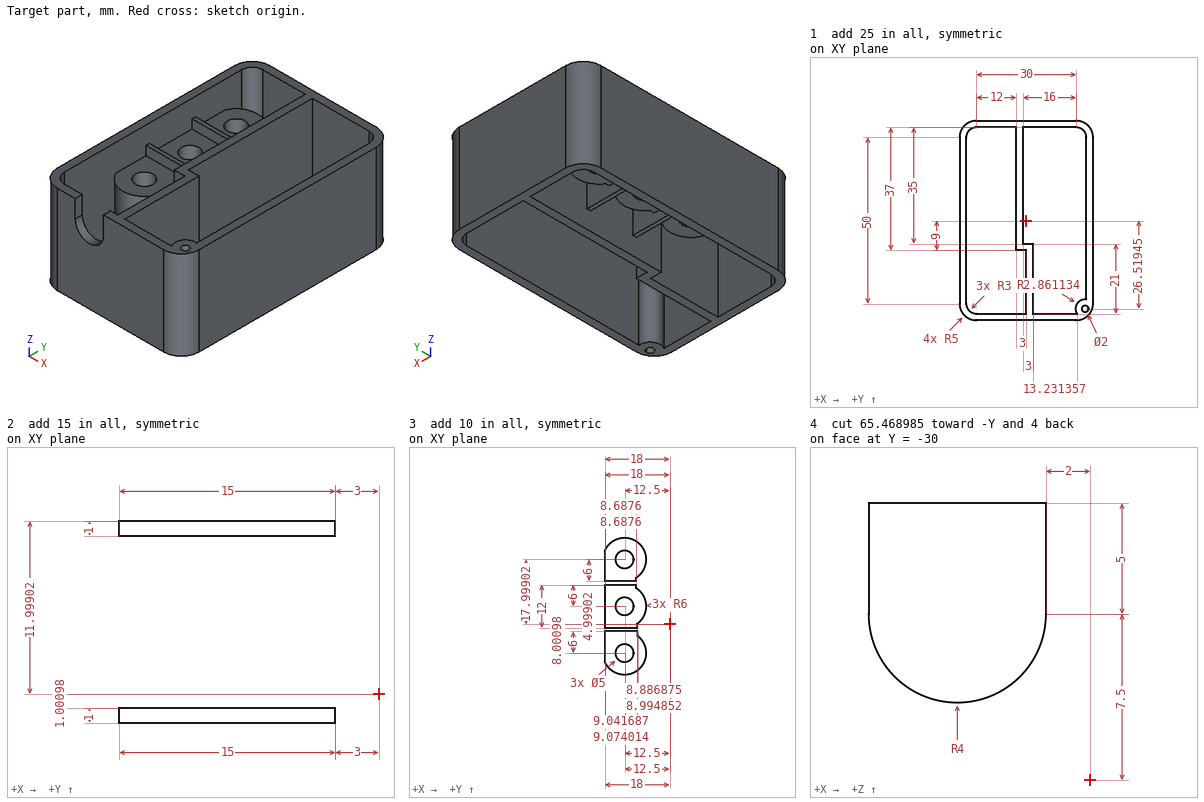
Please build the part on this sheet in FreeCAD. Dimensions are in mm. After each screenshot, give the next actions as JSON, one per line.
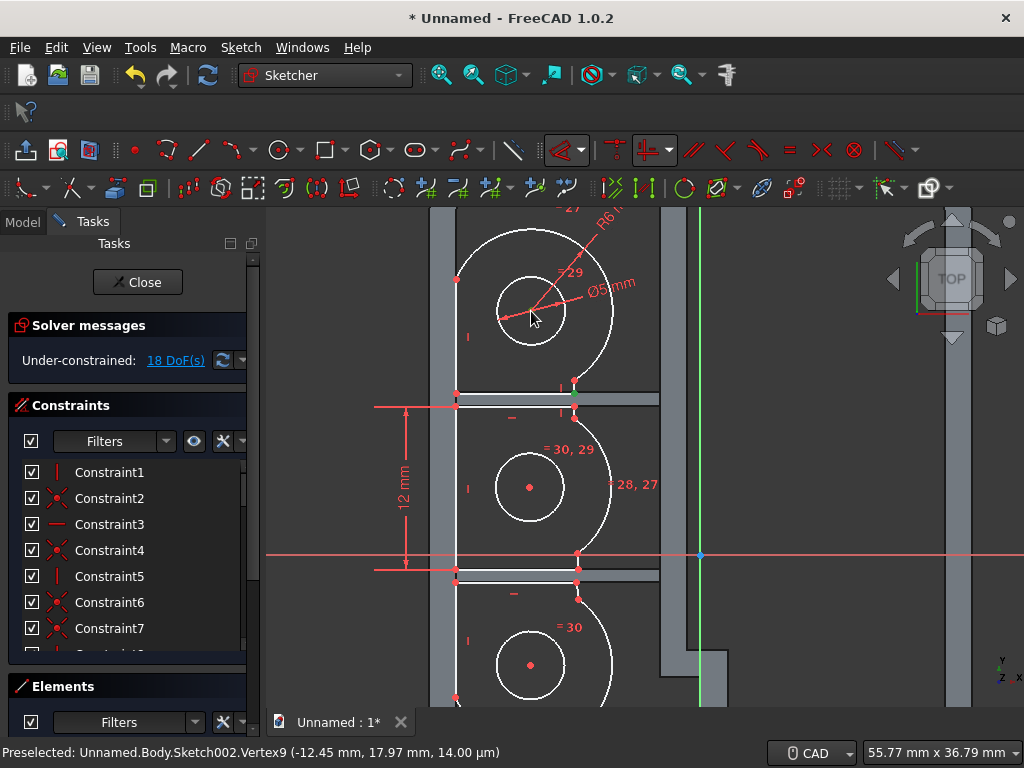
{"action": "left_click", "coordinate": [584, 150]}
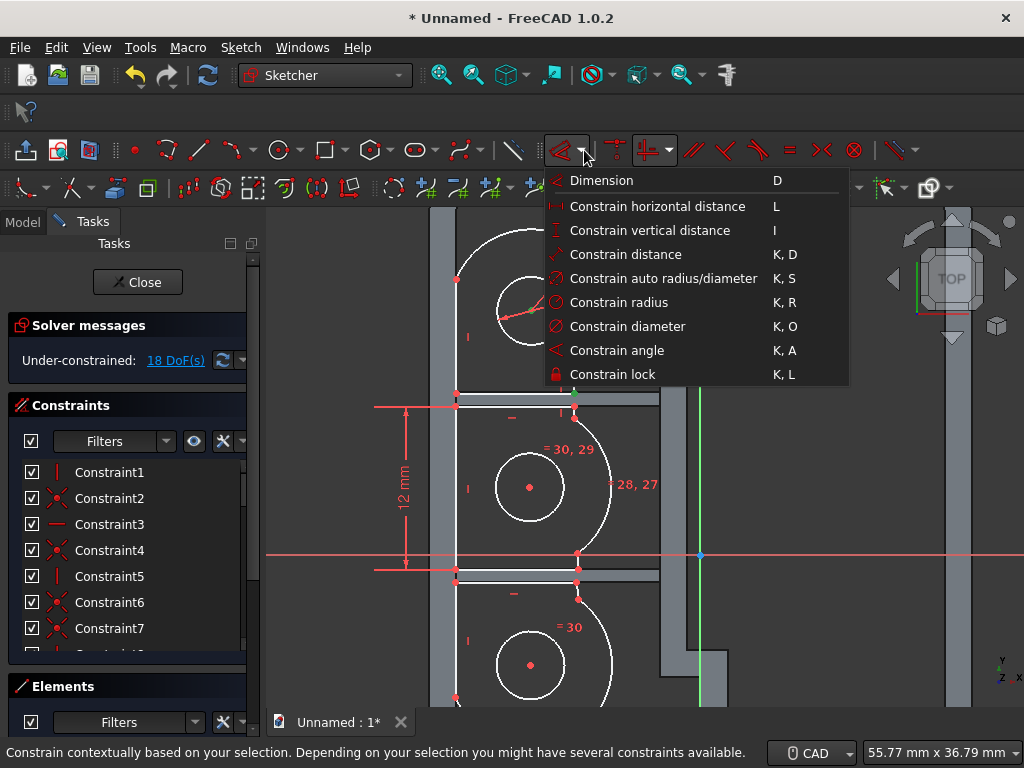
{"action": "left_click", "coordinate": [697, 230]}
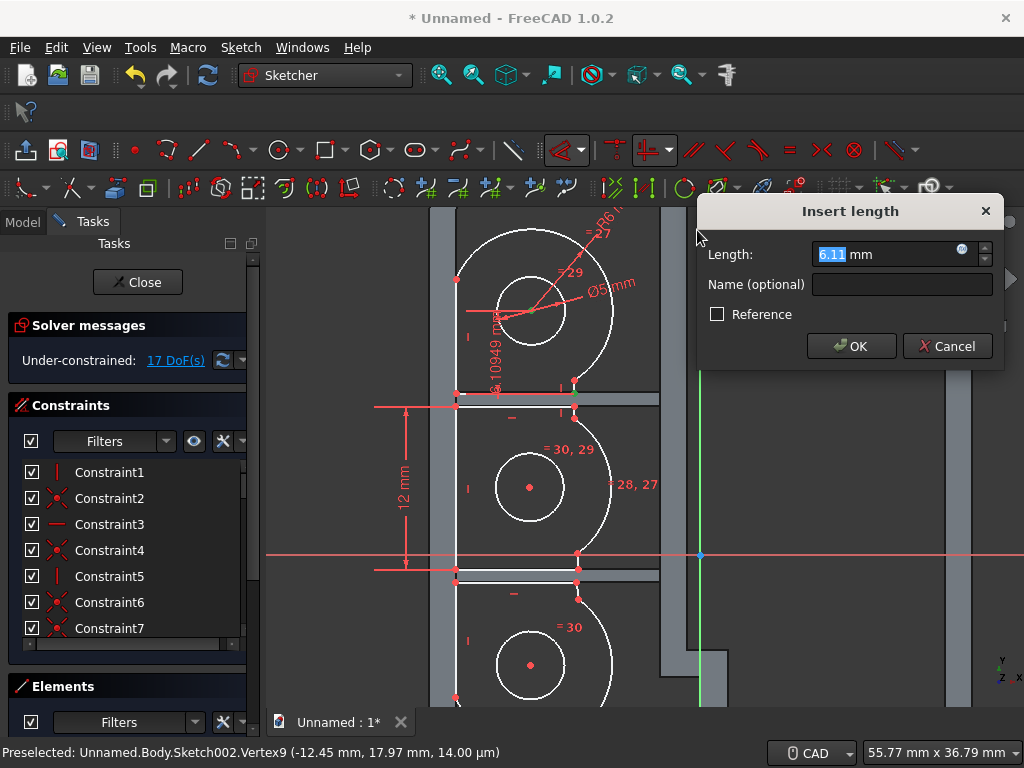
{"action": "type", "text": "6"}
{"action": "key", "text": "Return"}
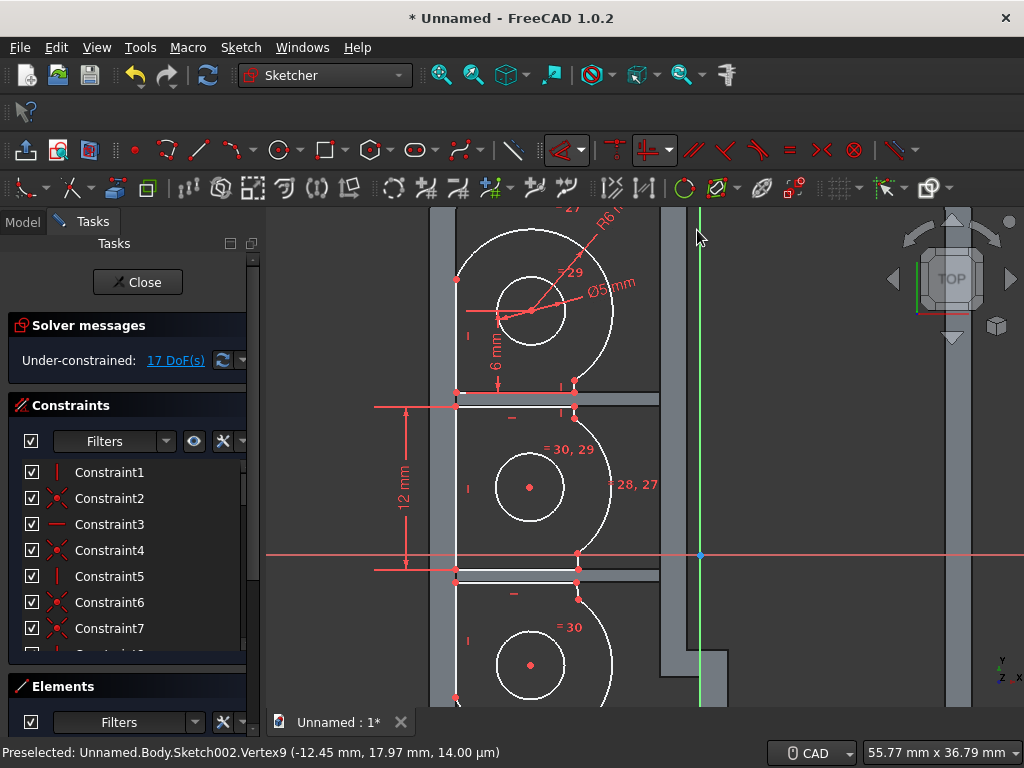
{"action": "left_click", "coordinate": [574, 407]}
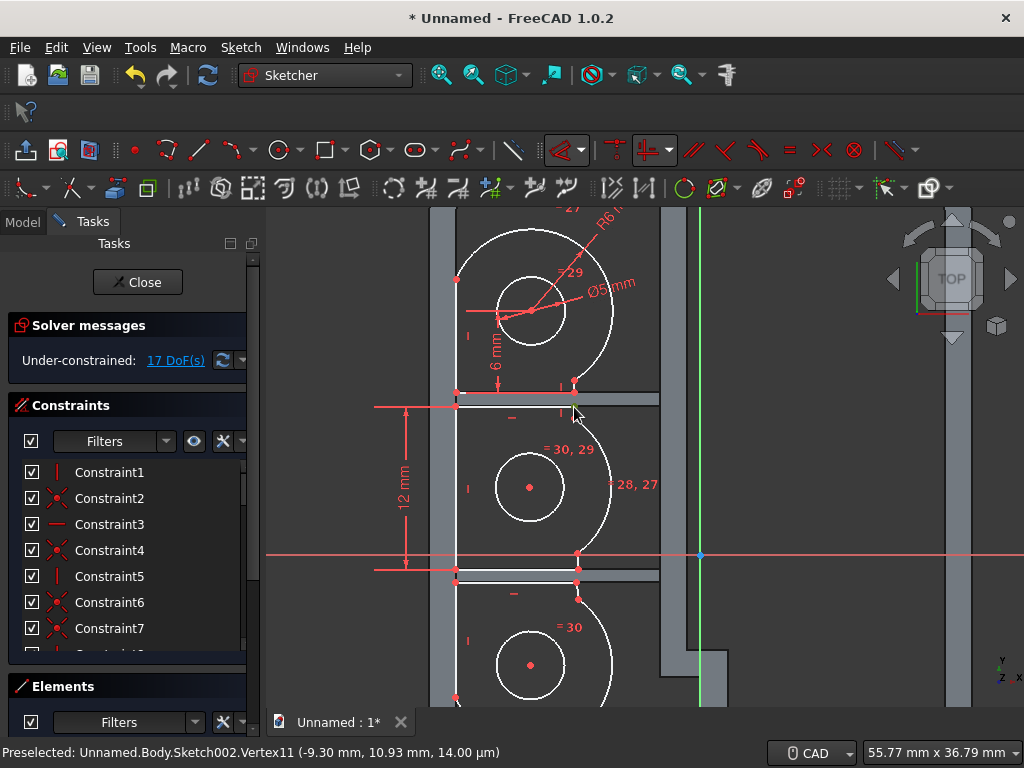
{"action": "left_click", "coordinate": [530, 487]}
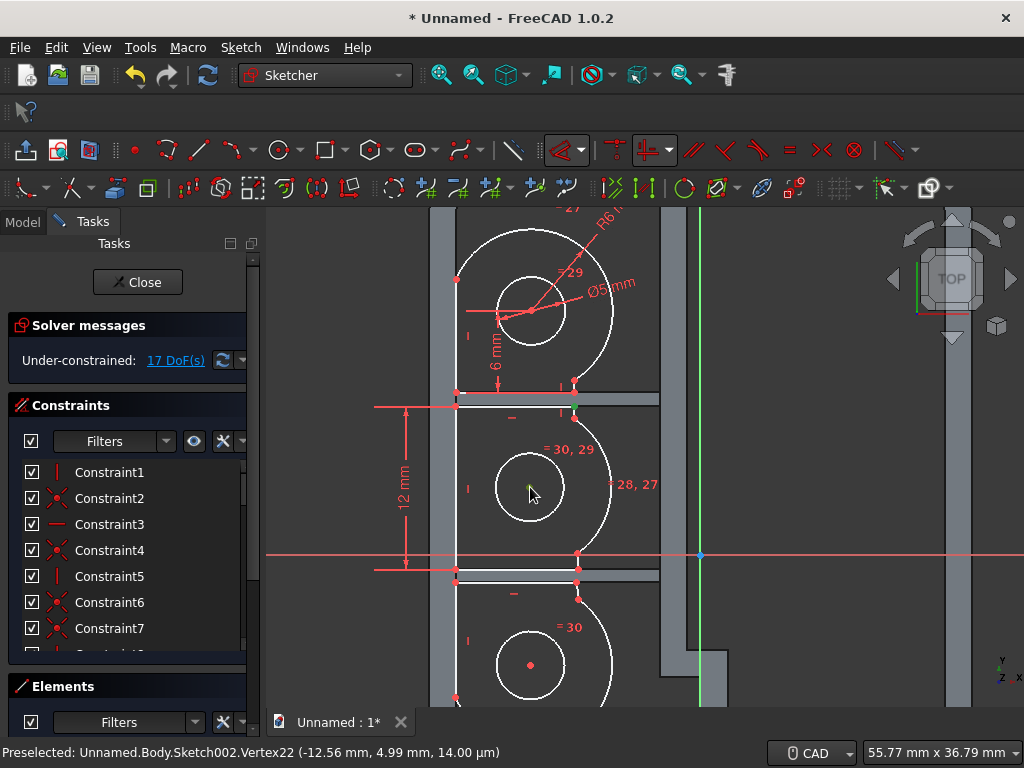
{"action": "left_click", "coordinate": [584, 150]}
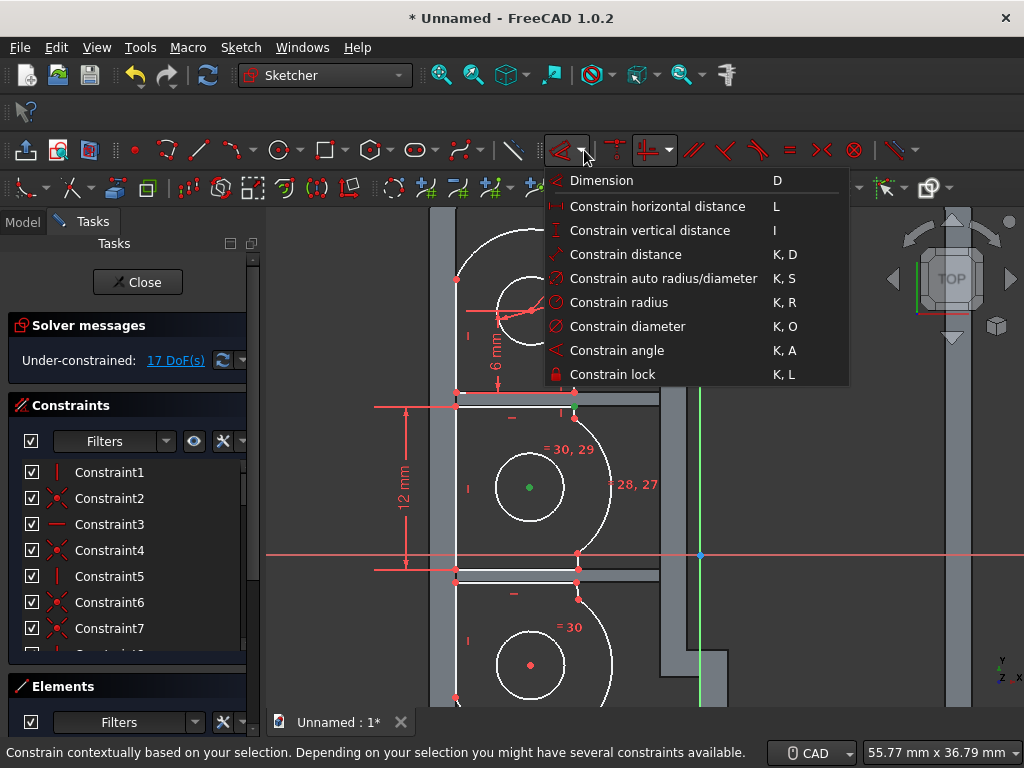
{"action": "left_click", "coordinate": [697, 230]}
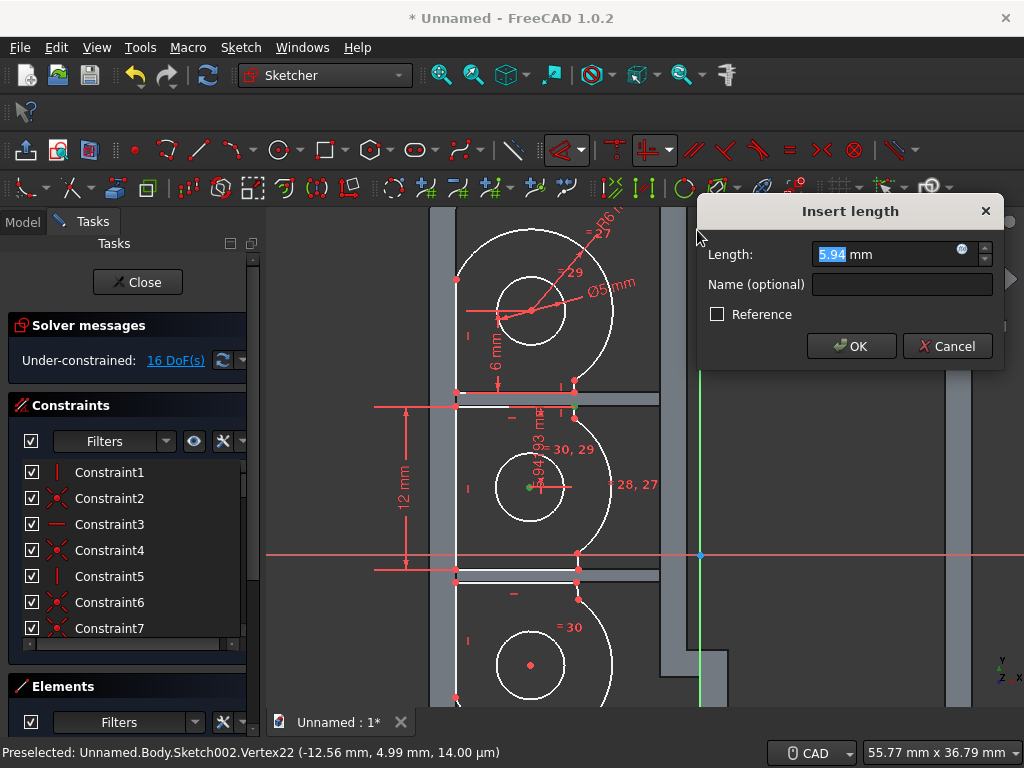
{"action": "type", "text": "6"}
{"action": "key", "text": "Return"}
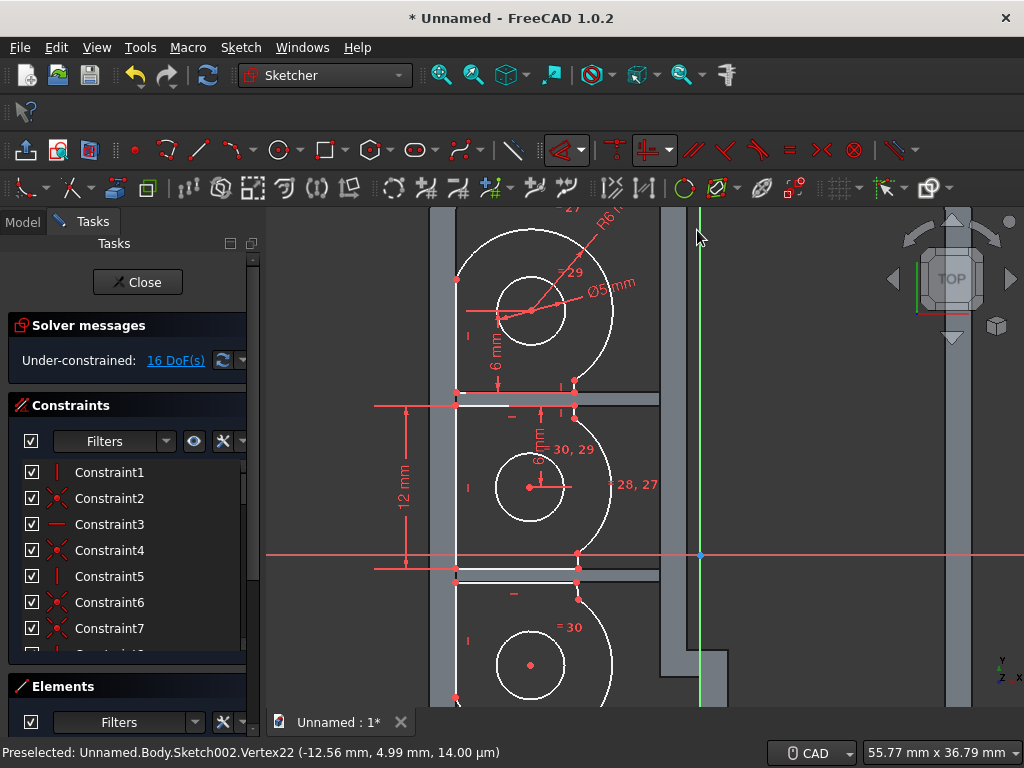
{"action": "left_click", "coordinate": [577, 583]}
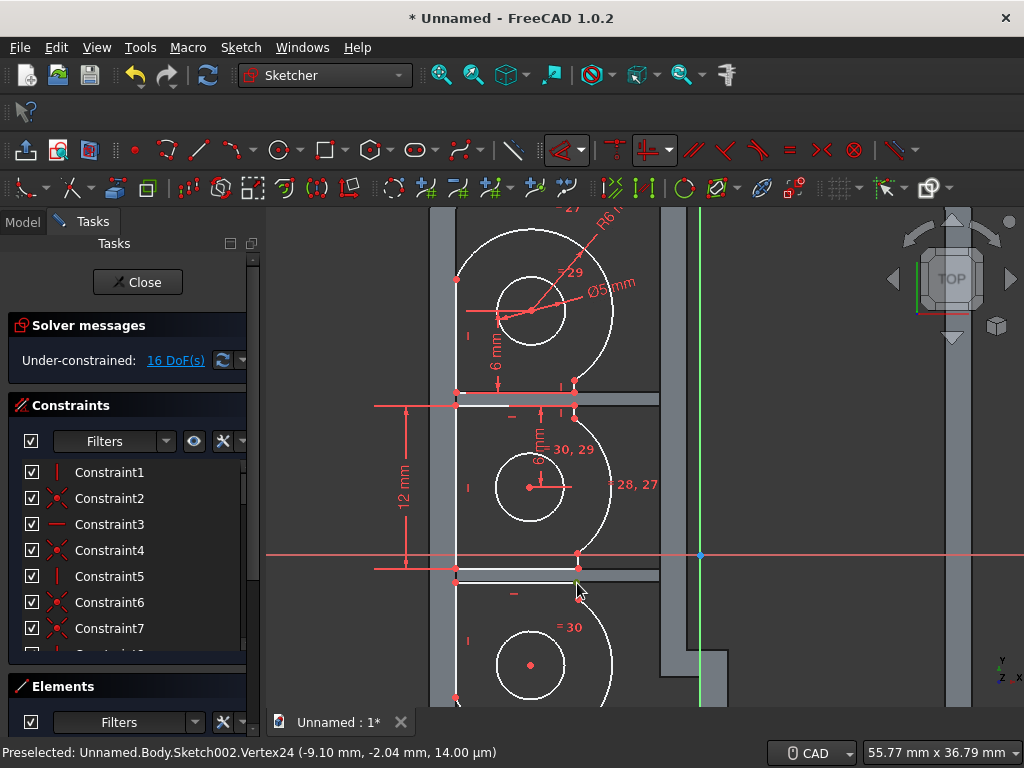
{"action": "left_click", "coordinate": [531, 665]}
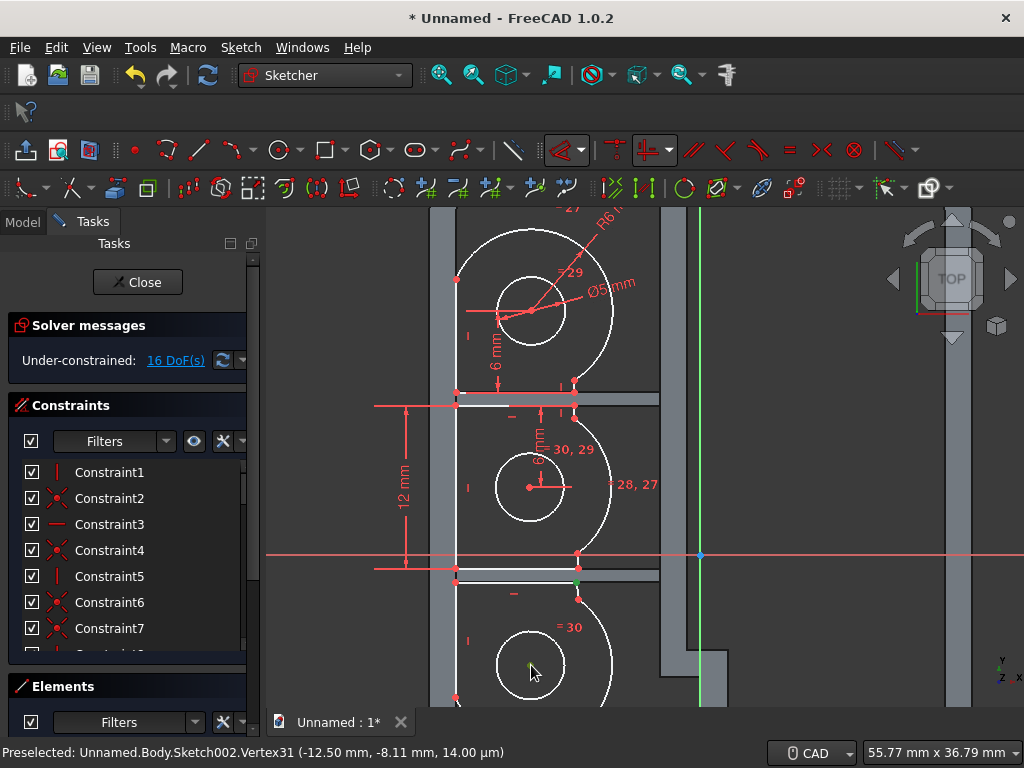
{"action": "key", "text": "i"}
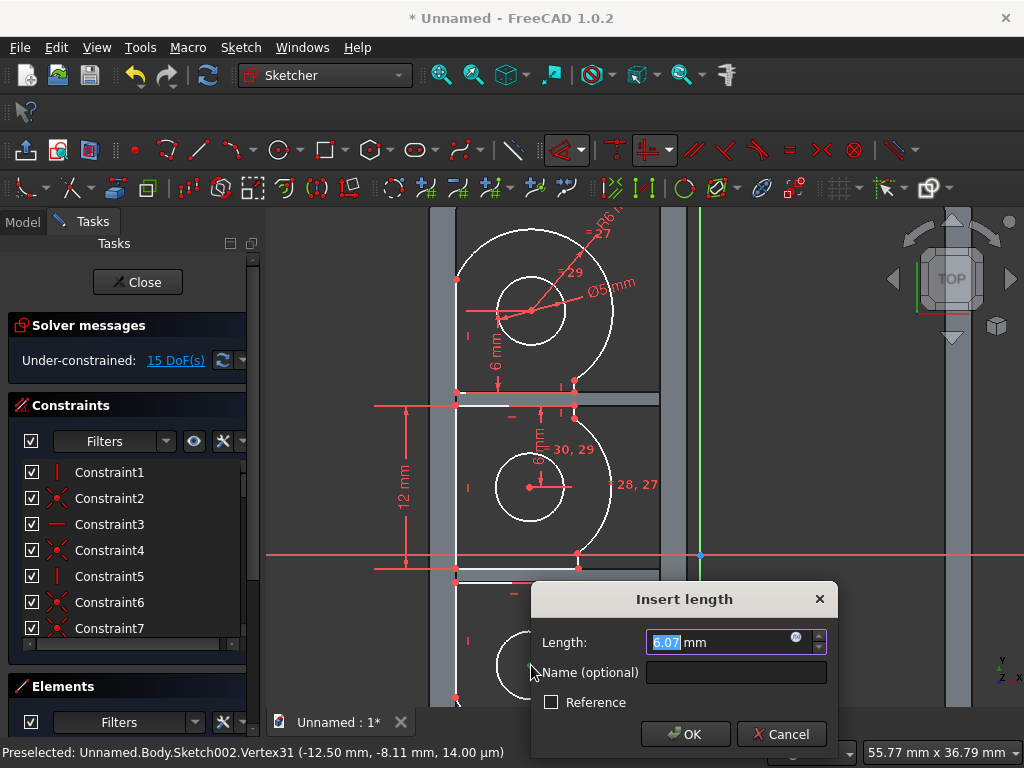
{"action": "type", "text": "6"}
{"action": "key", "text": "Return"}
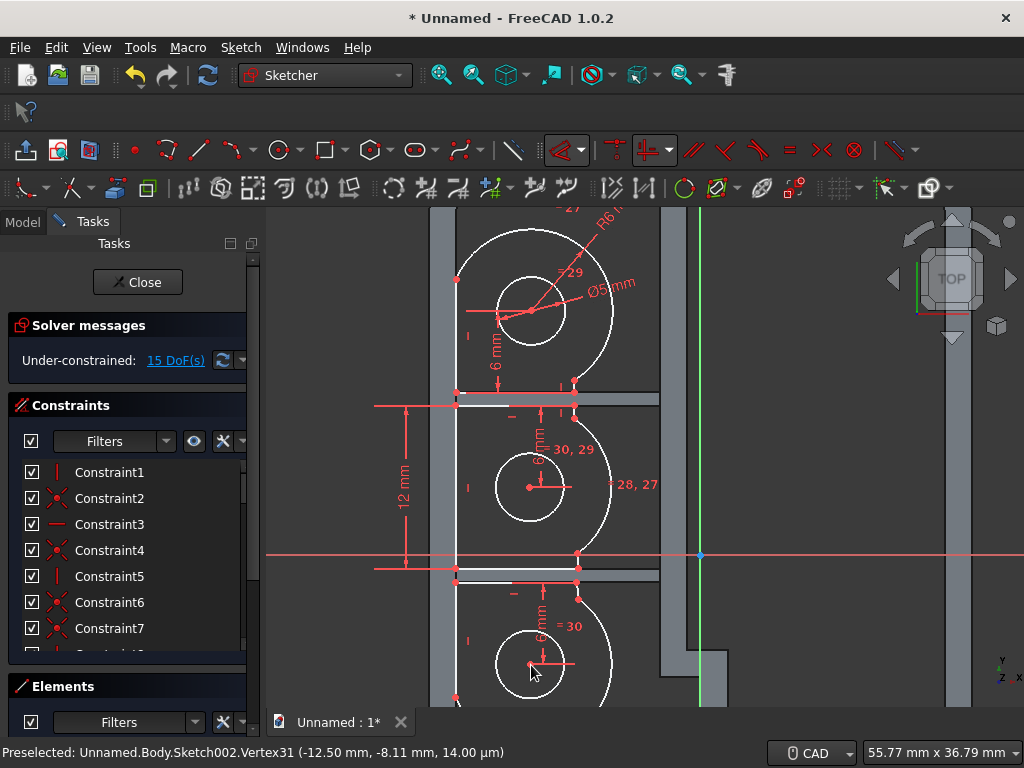
{"action": "left_click", "coordinate": [456, 279]}